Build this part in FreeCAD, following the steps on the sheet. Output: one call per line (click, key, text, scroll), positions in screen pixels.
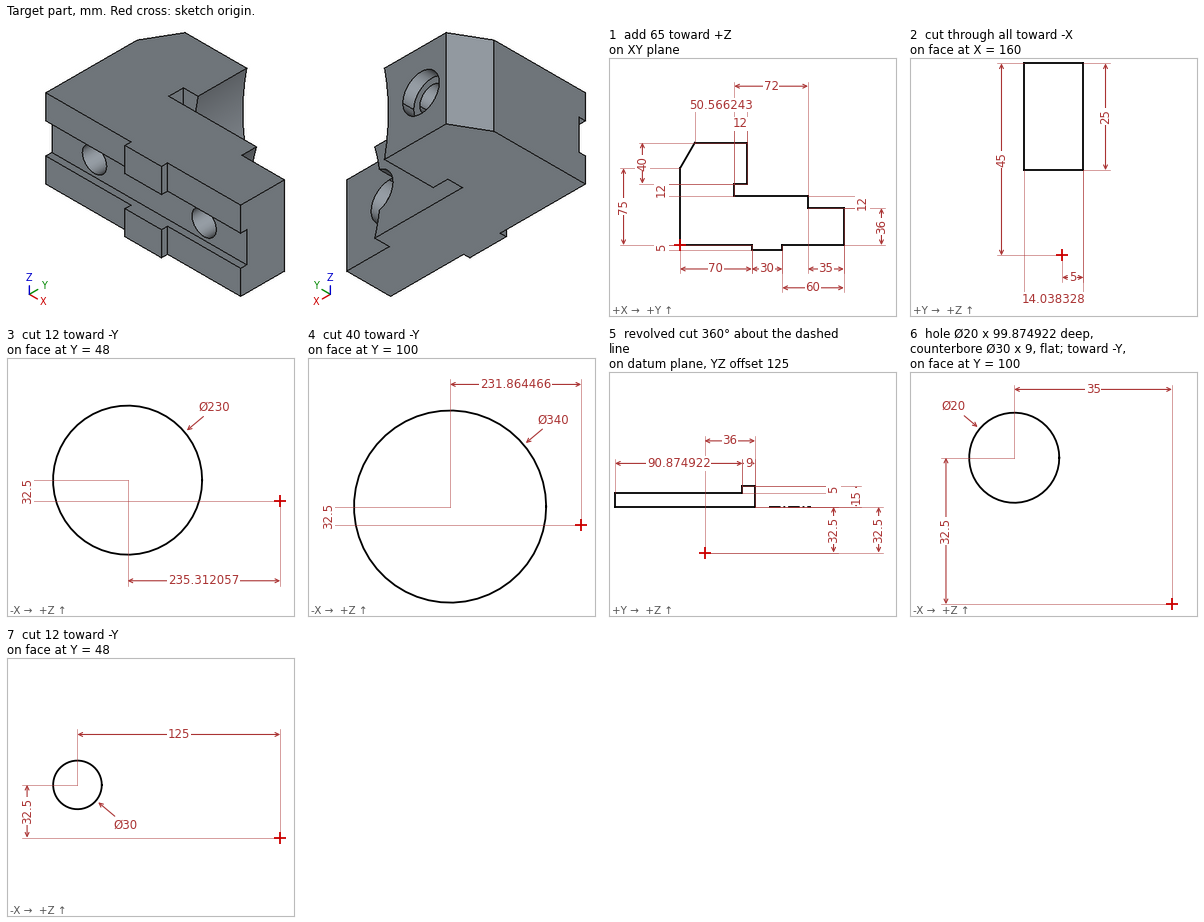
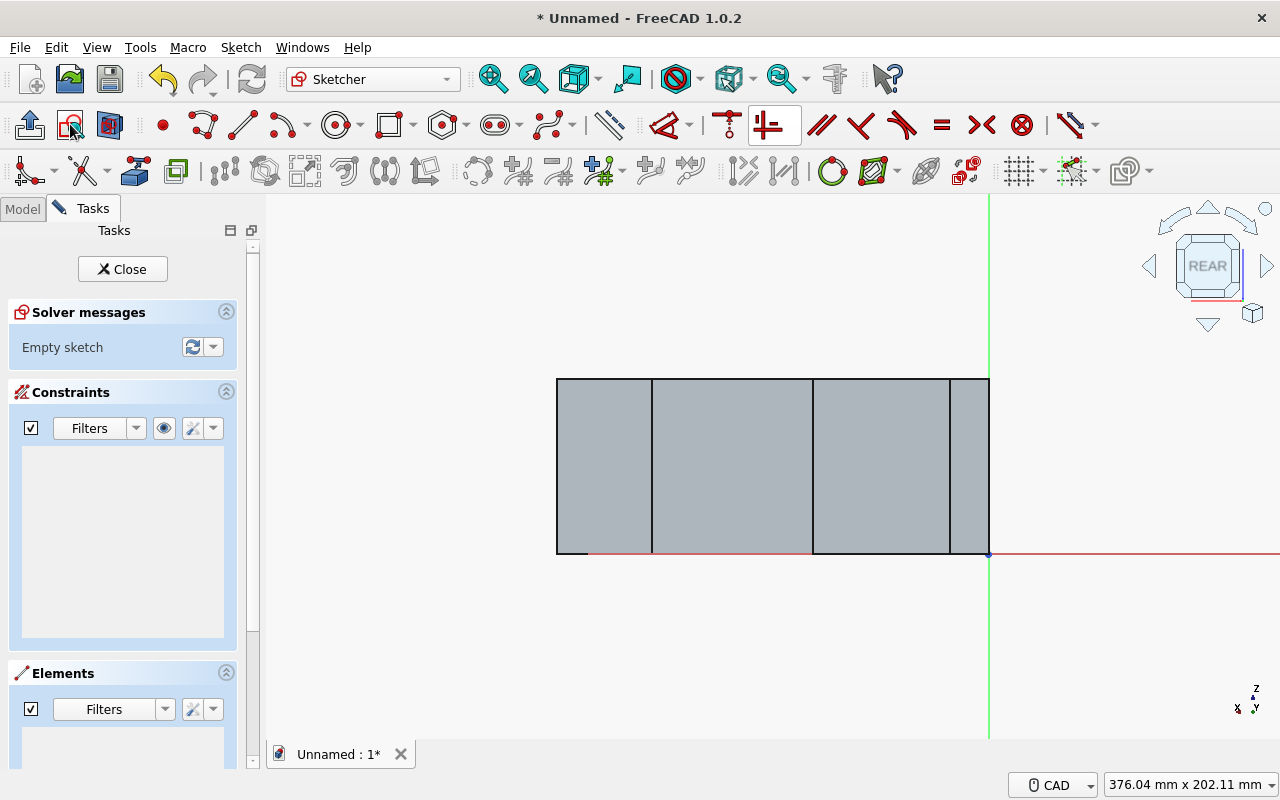
scroll(933, 466, down, 3)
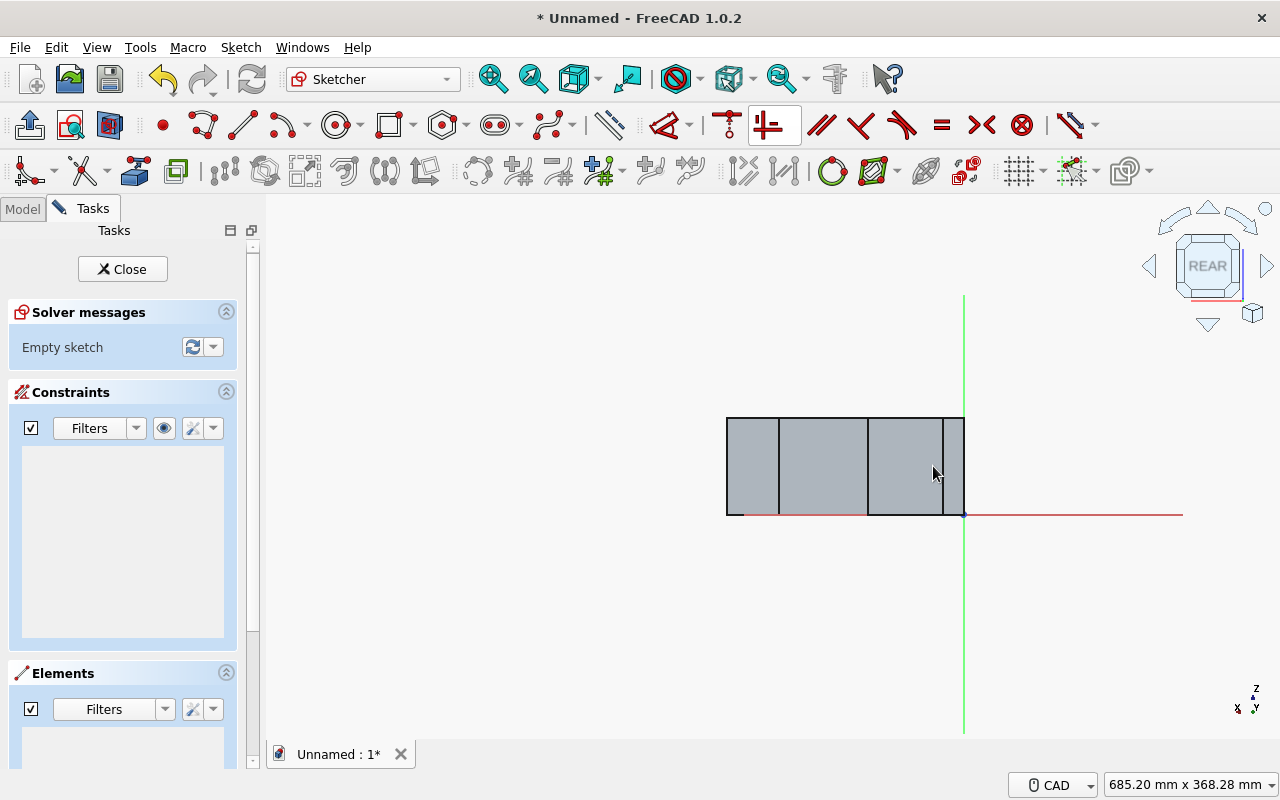
click(336, 126)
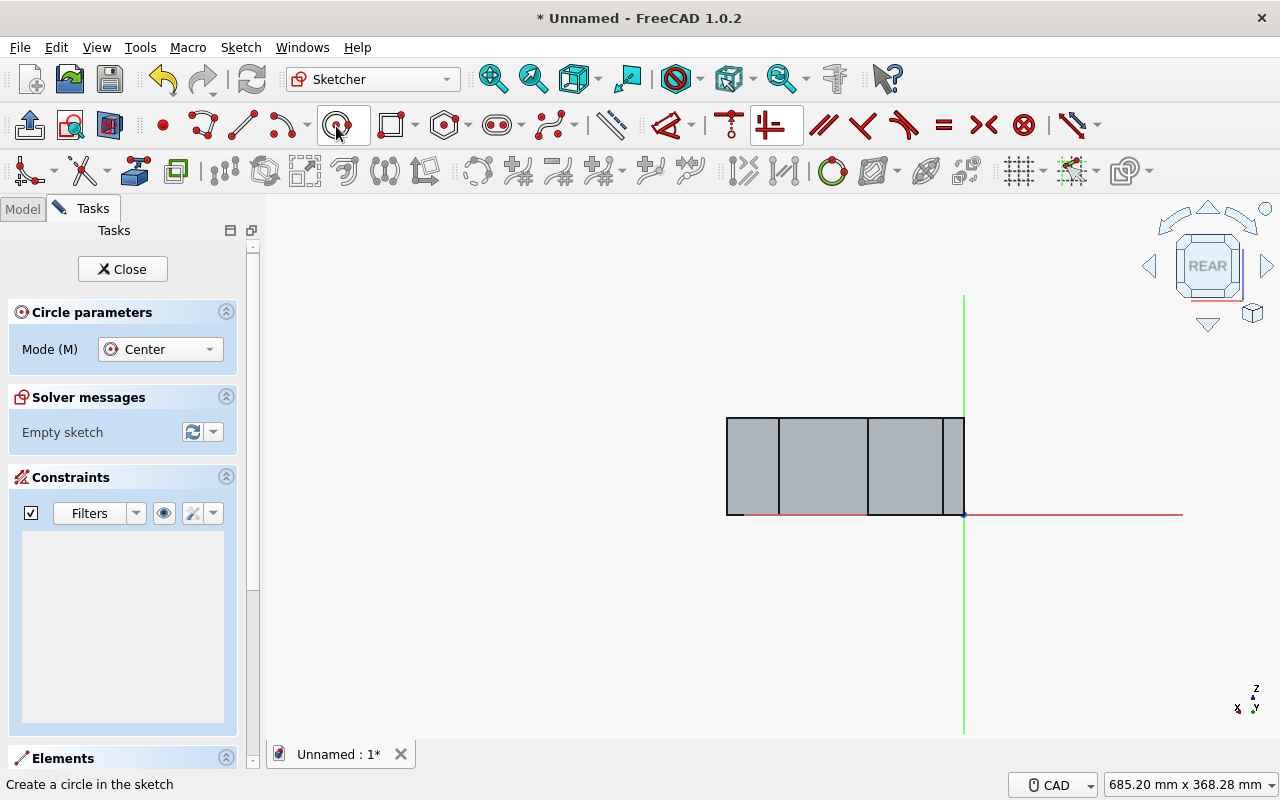
click(616, 466)
move(736, 346)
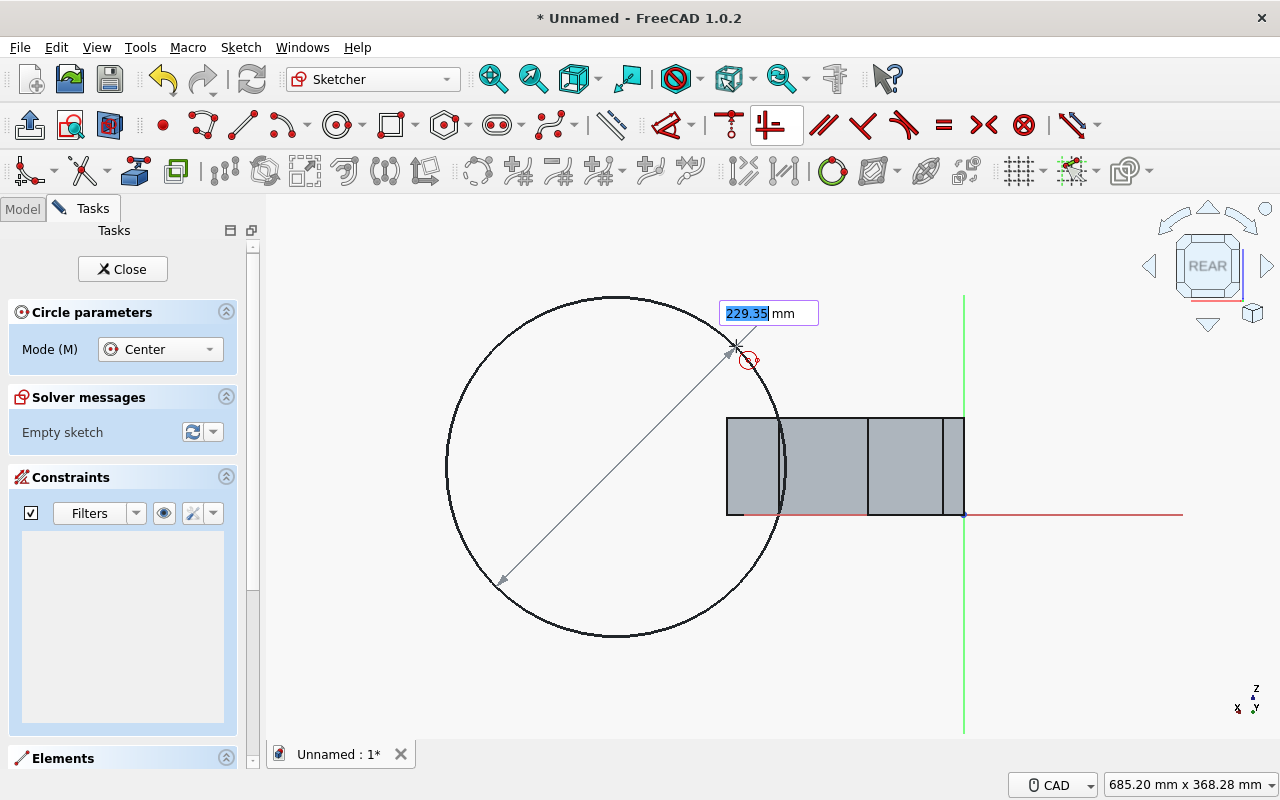
text(230)
key(Return)
key(Escape)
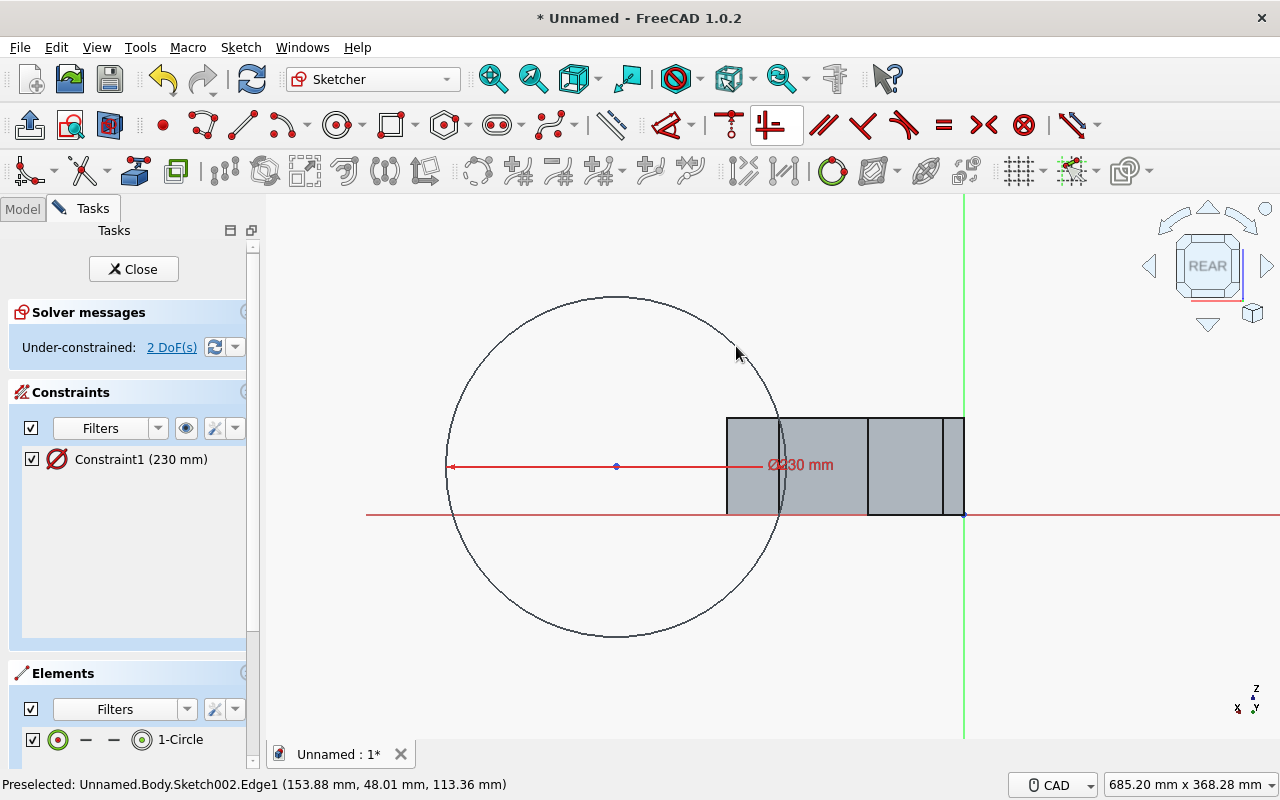
click(666, 126)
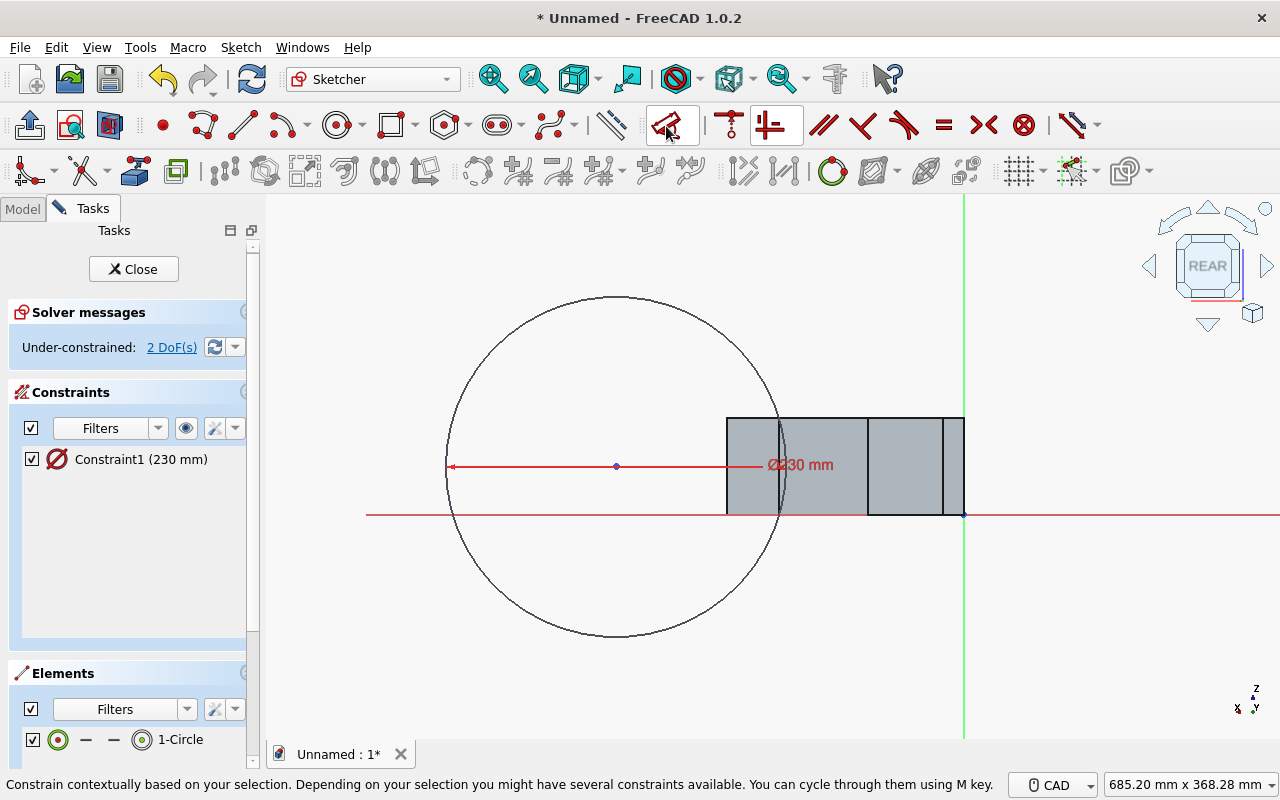
click(616, 467)
click(998, 491)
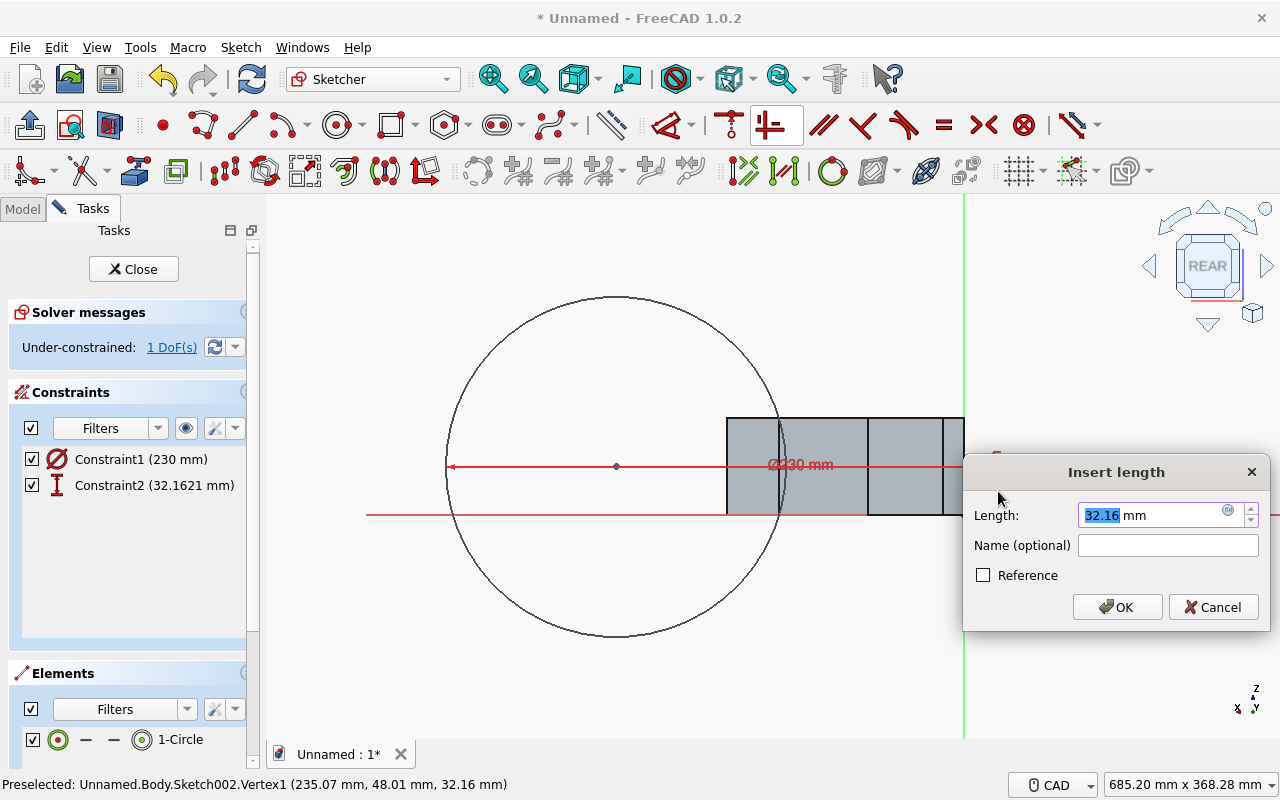
text(32.5)
key(Return)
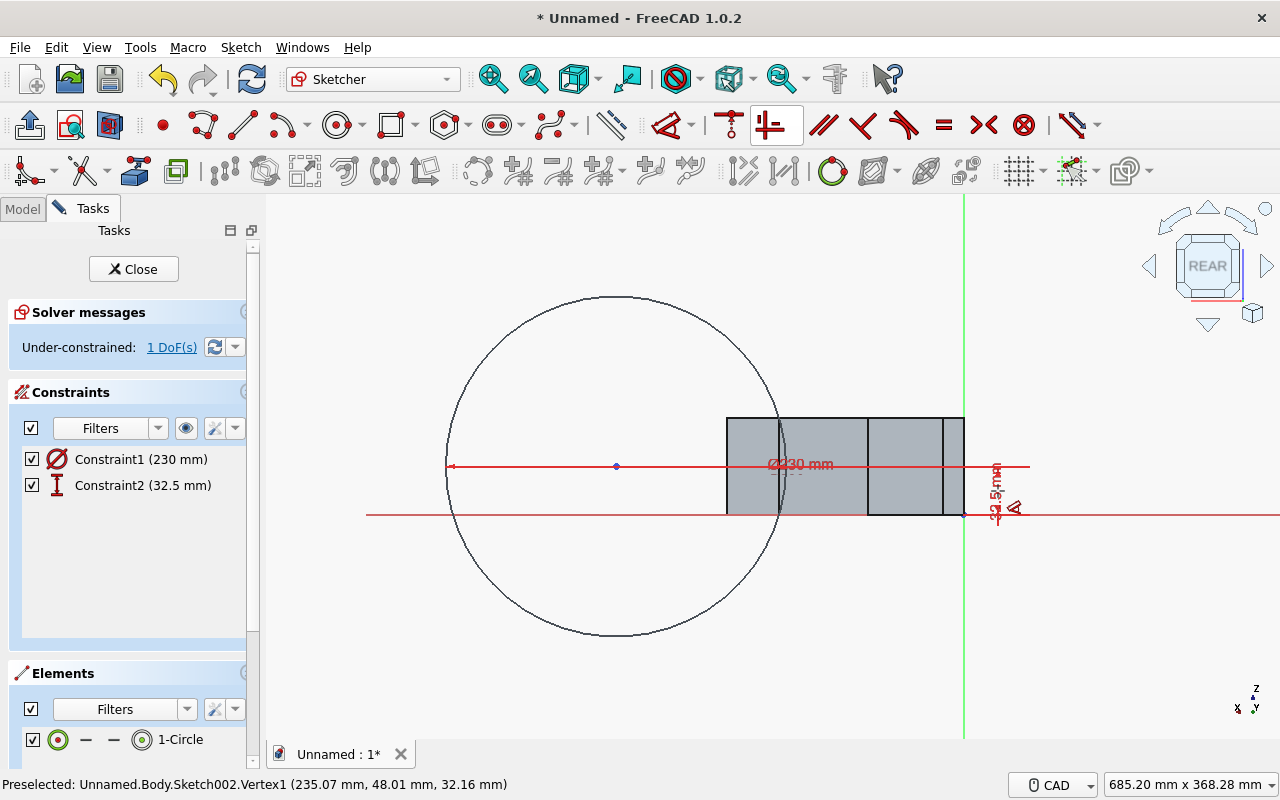
click(616, 466)
click(790, 549)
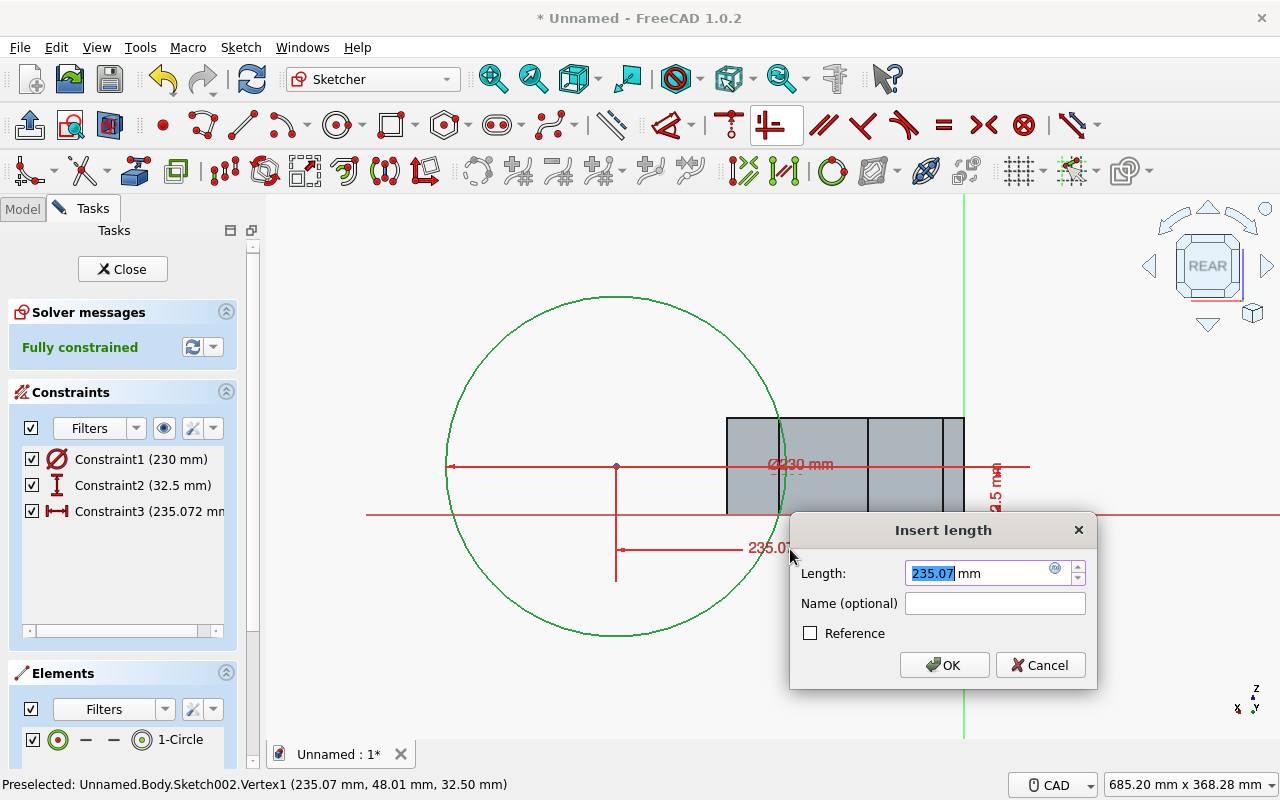
text(235.312057)
key(Return)
key(Escape)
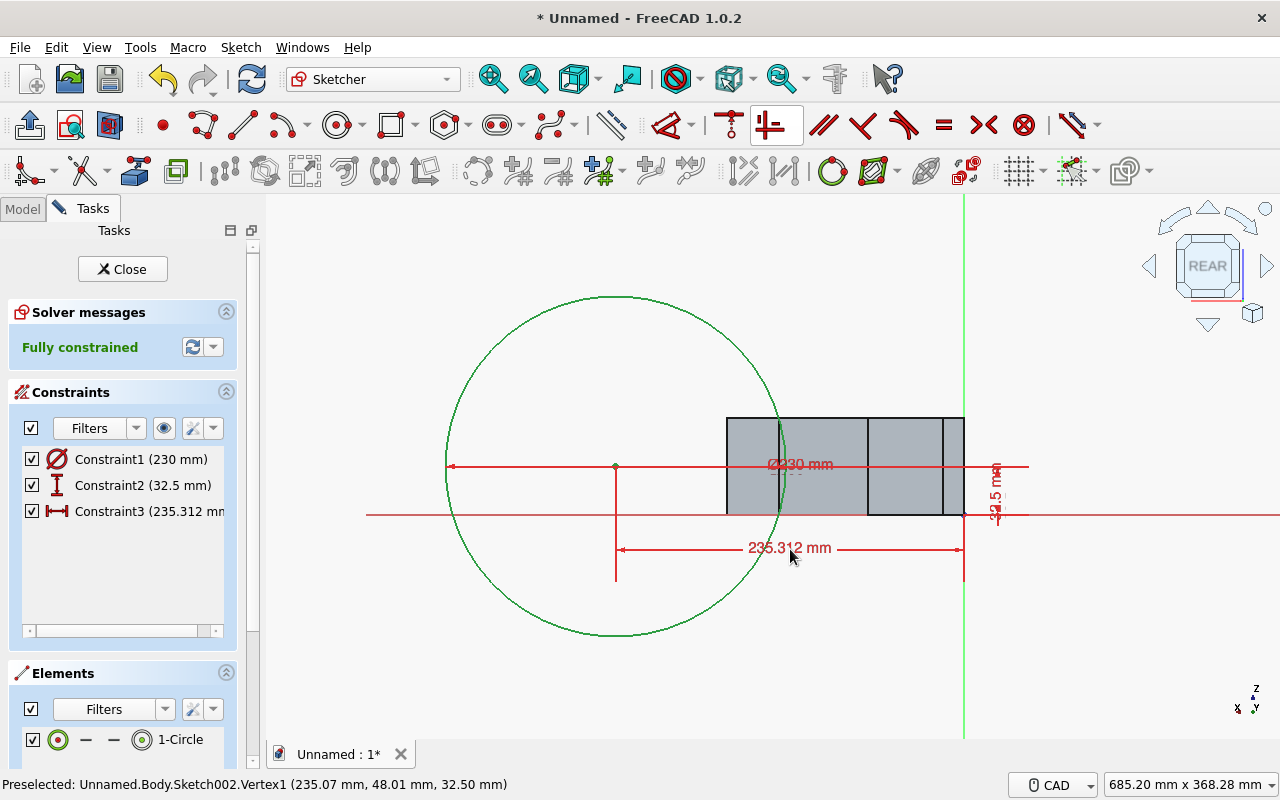
click(123, 269)